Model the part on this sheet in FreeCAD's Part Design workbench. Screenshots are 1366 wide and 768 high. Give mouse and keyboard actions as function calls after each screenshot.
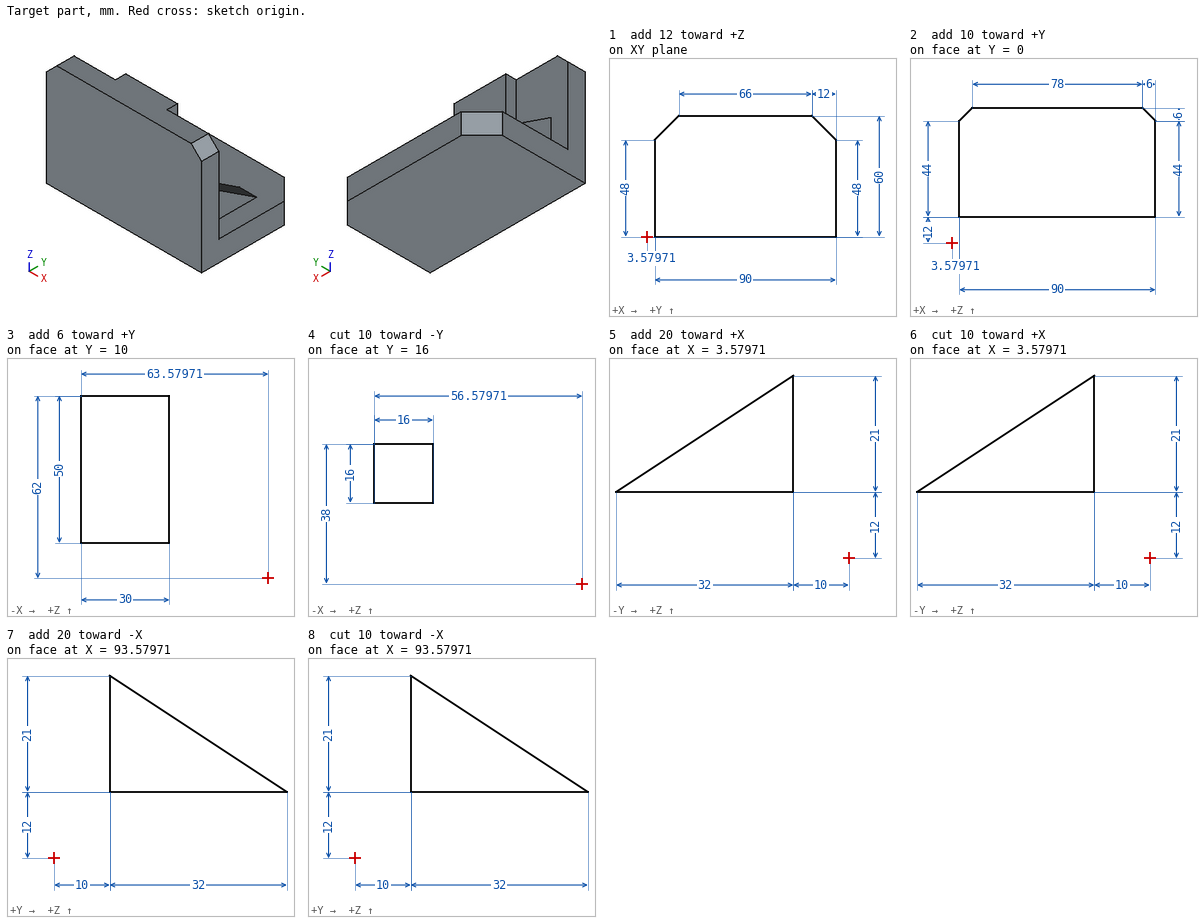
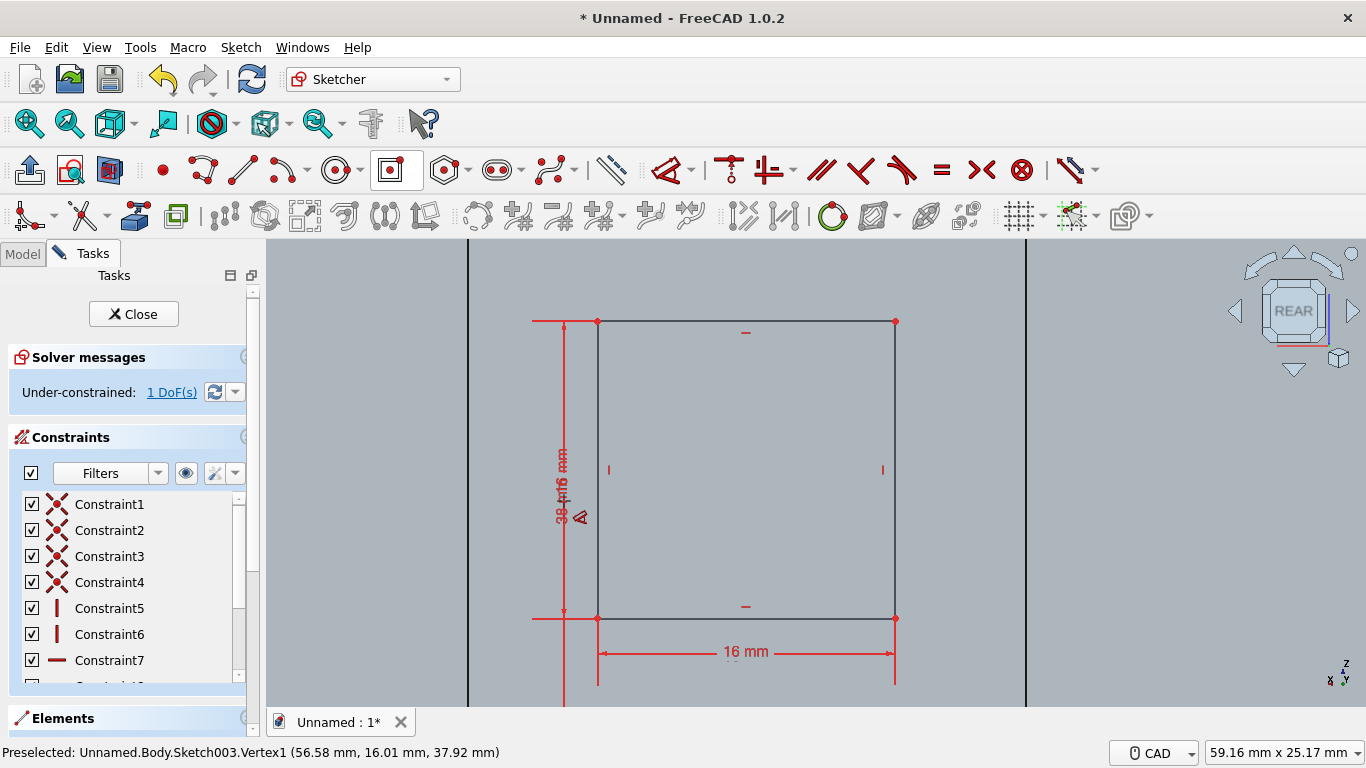
click(598, 321)
click(899, 287)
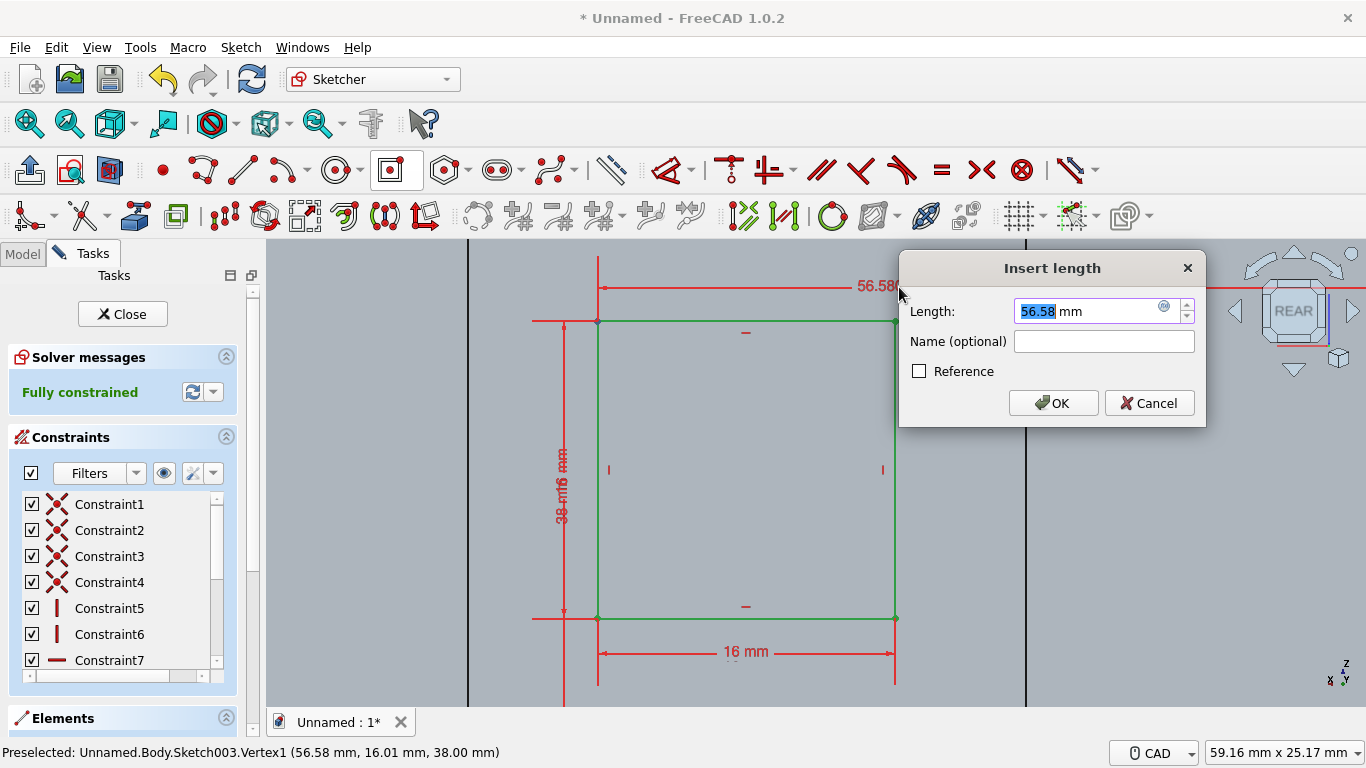
text(56.57971)
key(Return)
key(Escape)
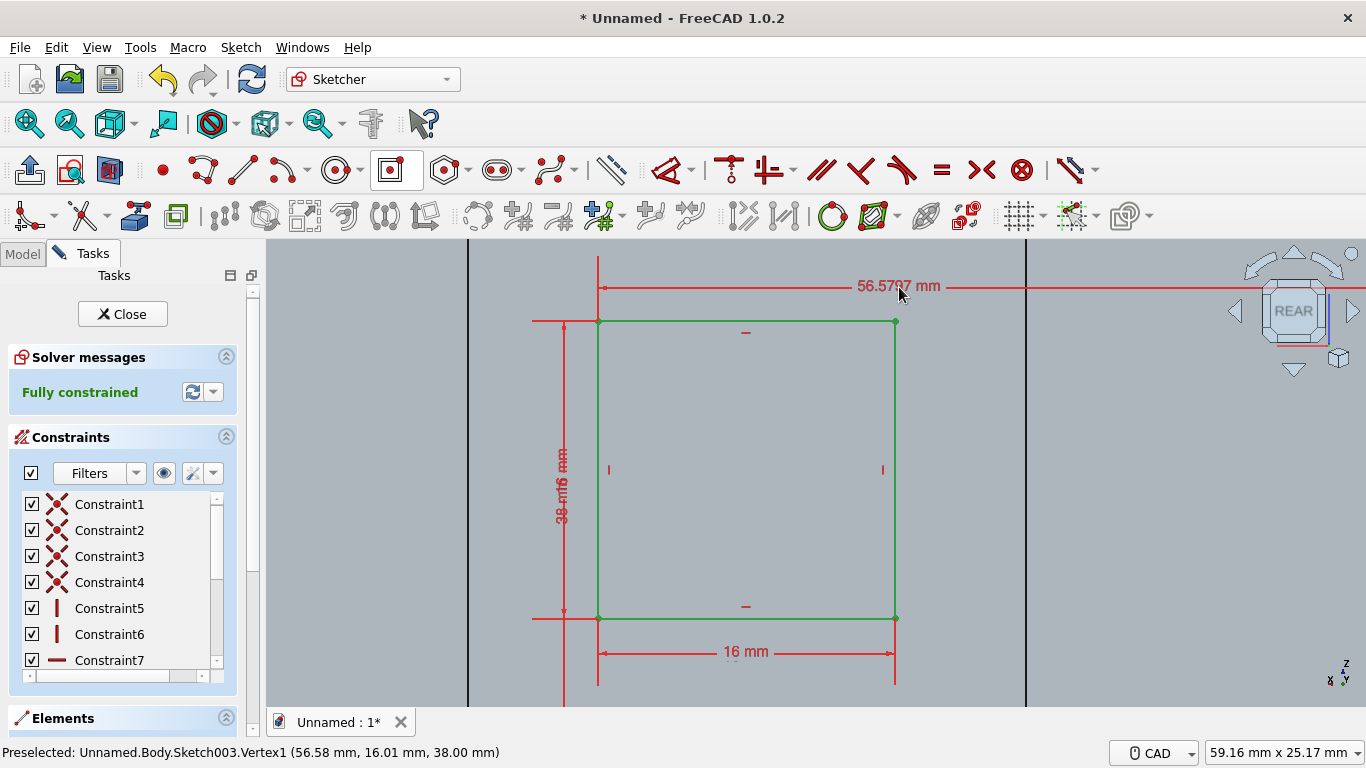
click(123, 314)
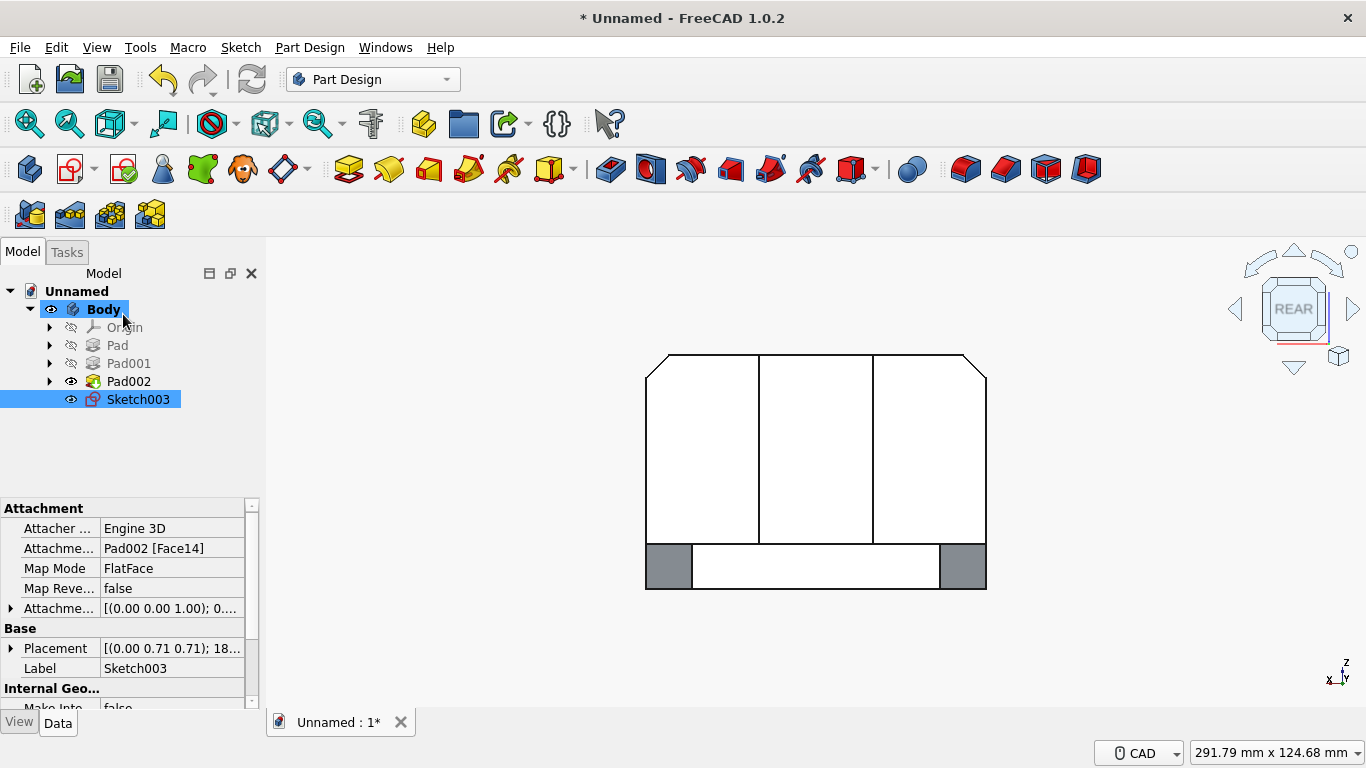
click(612, 170)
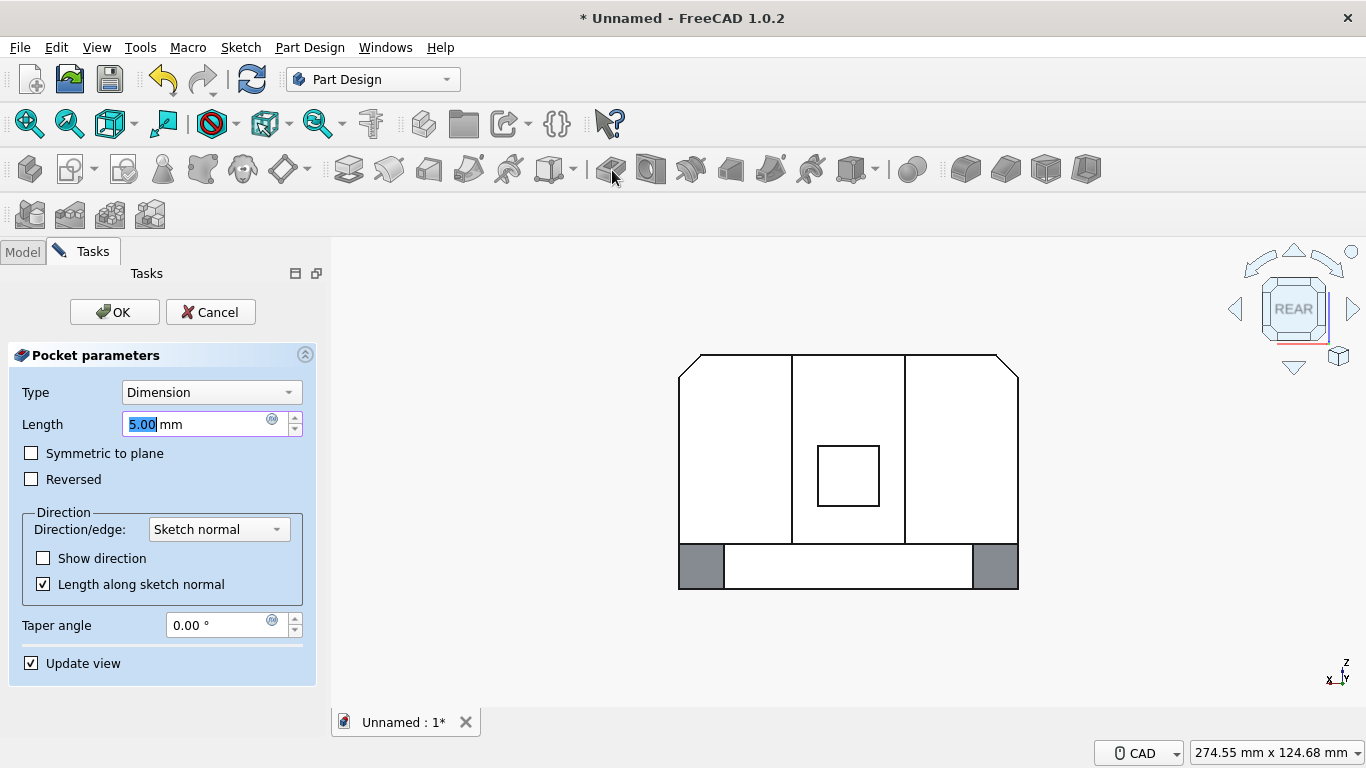
text(10)
key(Tab)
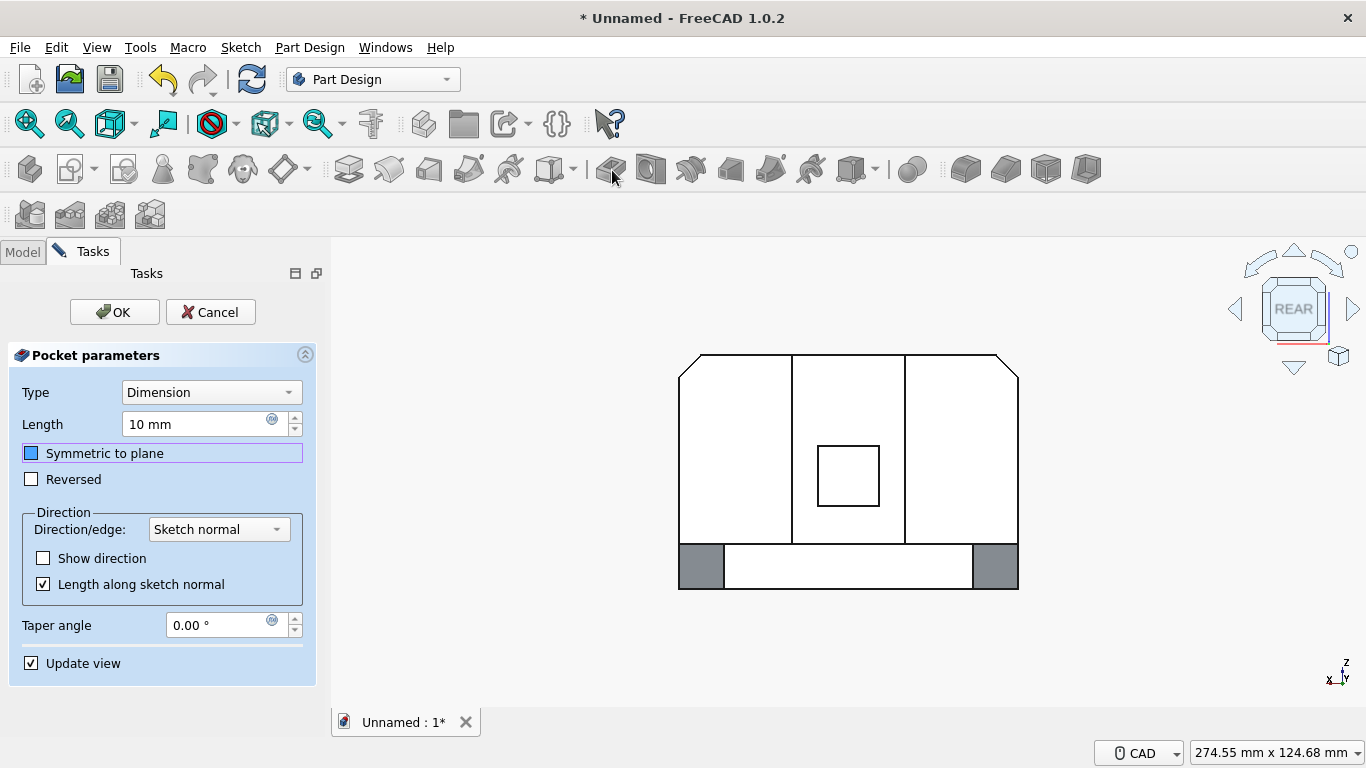
click(115, 312)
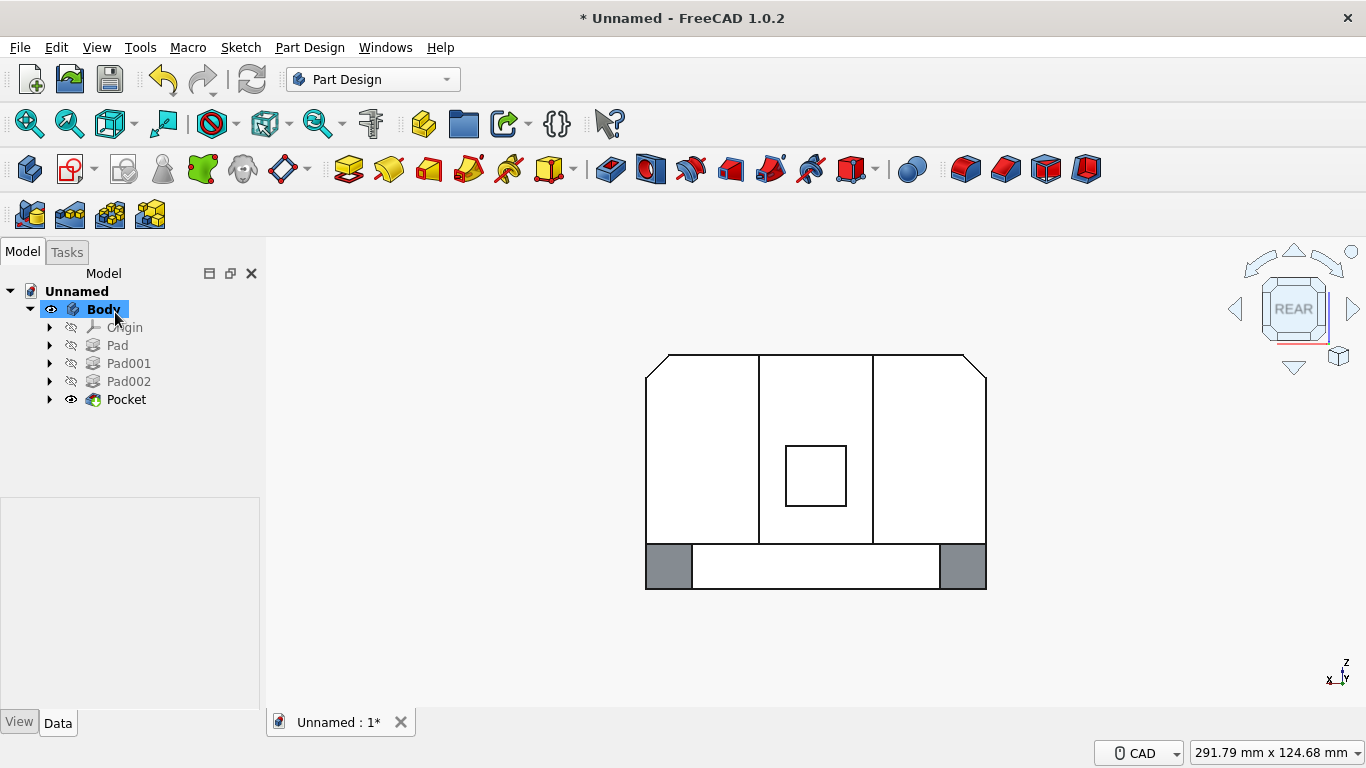
key(6)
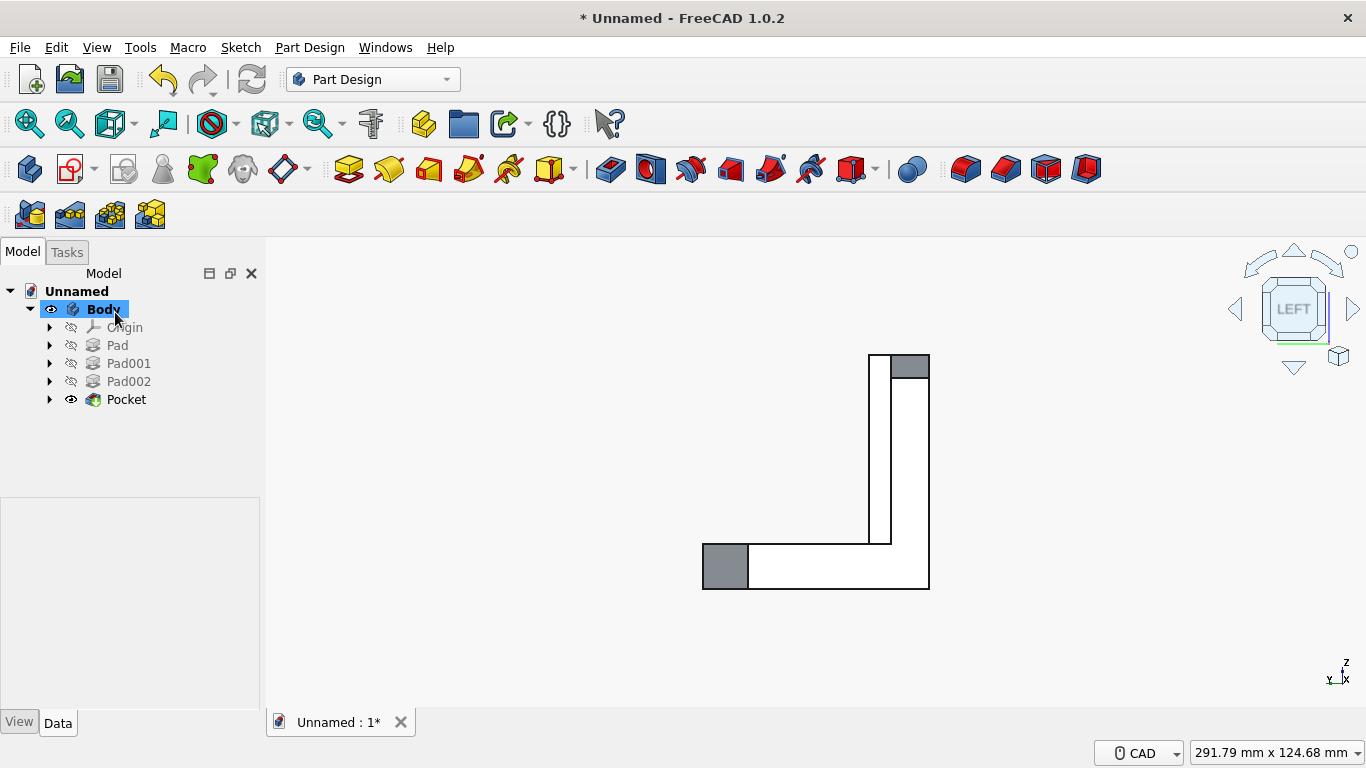
click(787, 573)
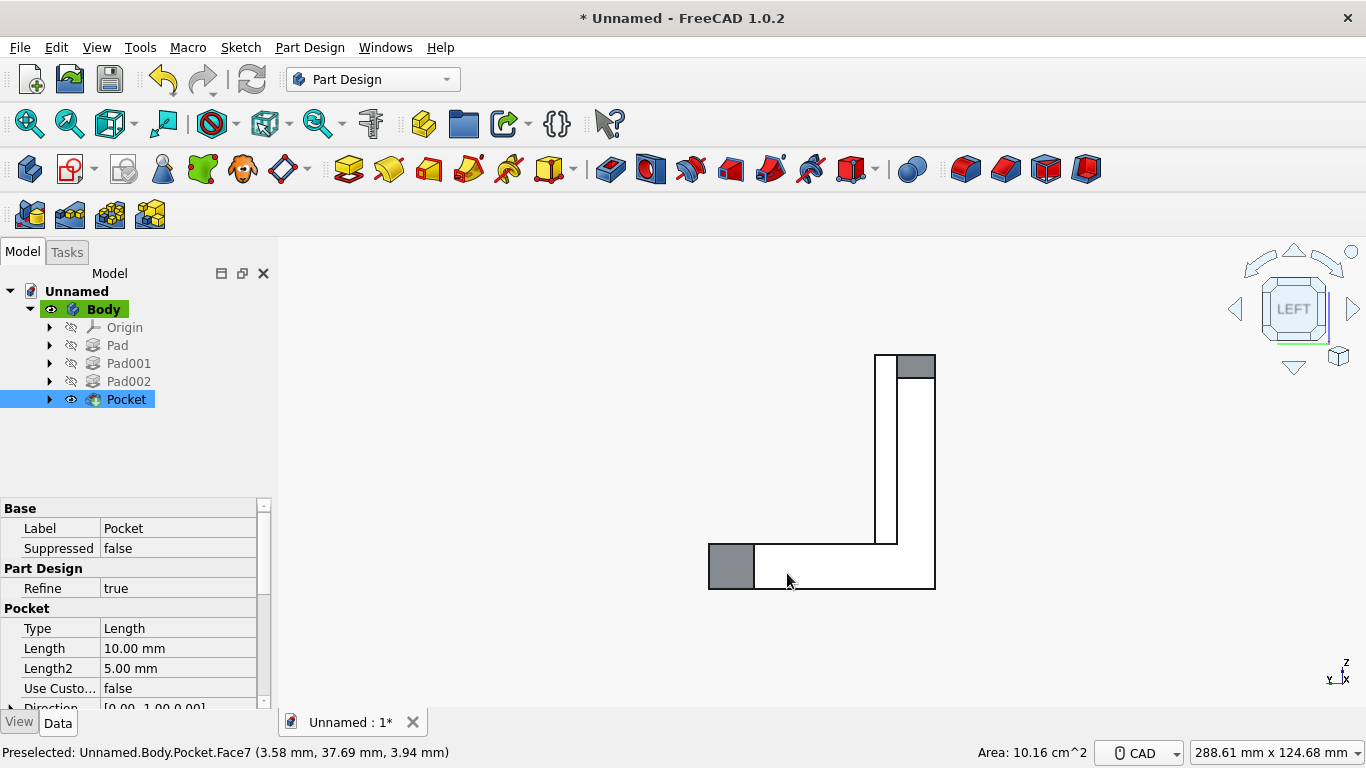
click(70, 170)